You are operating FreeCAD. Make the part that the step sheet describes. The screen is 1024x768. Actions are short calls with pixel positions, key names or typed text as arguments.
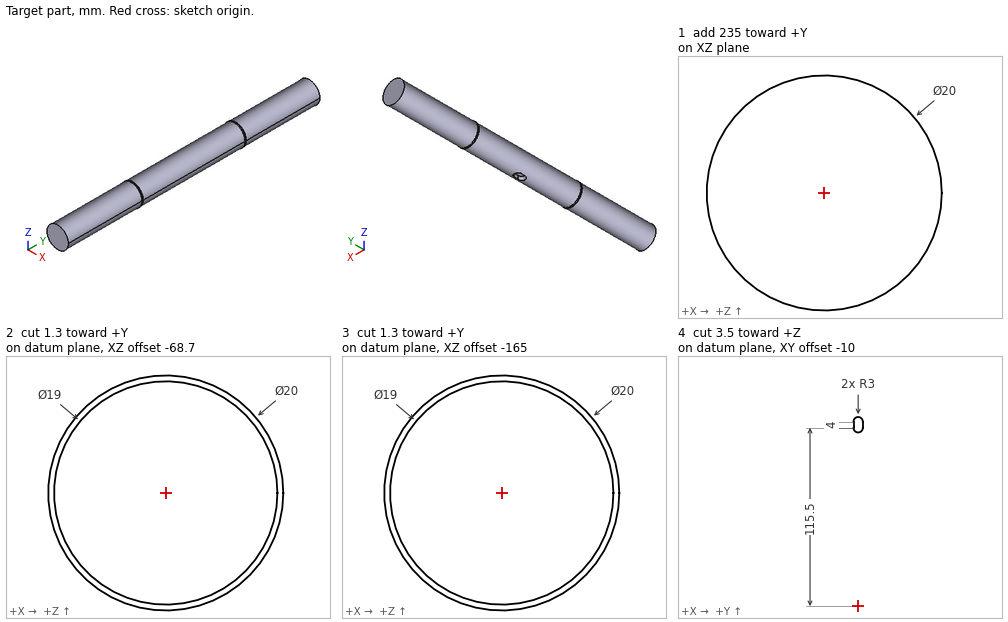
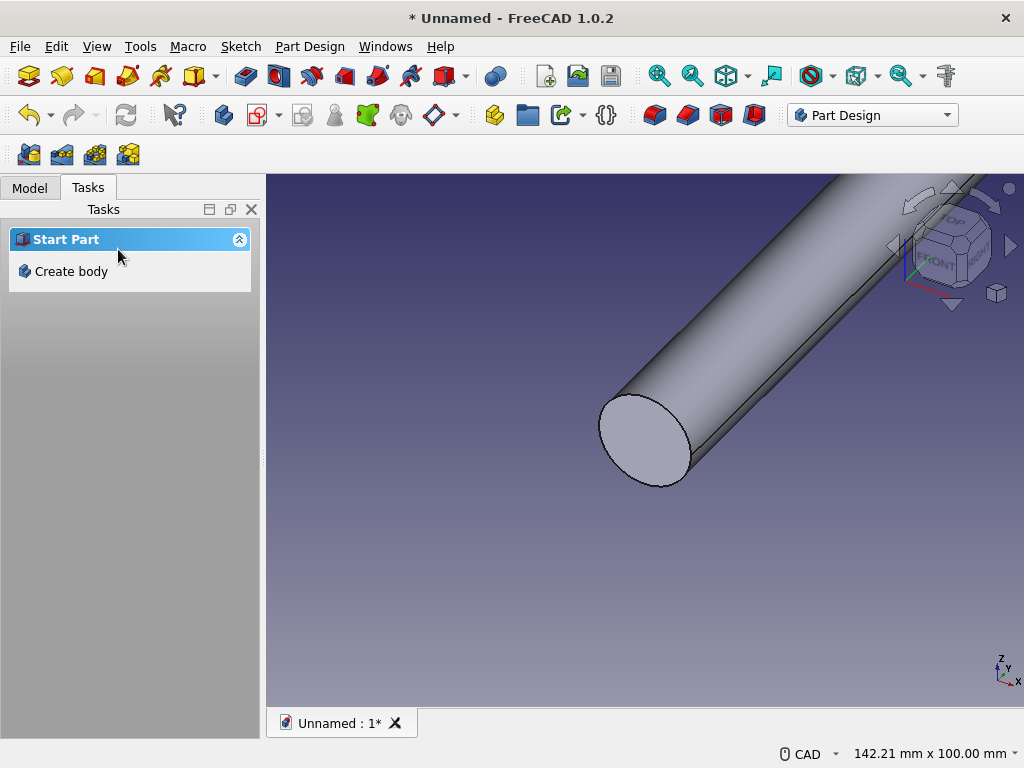
key(v)
key(f)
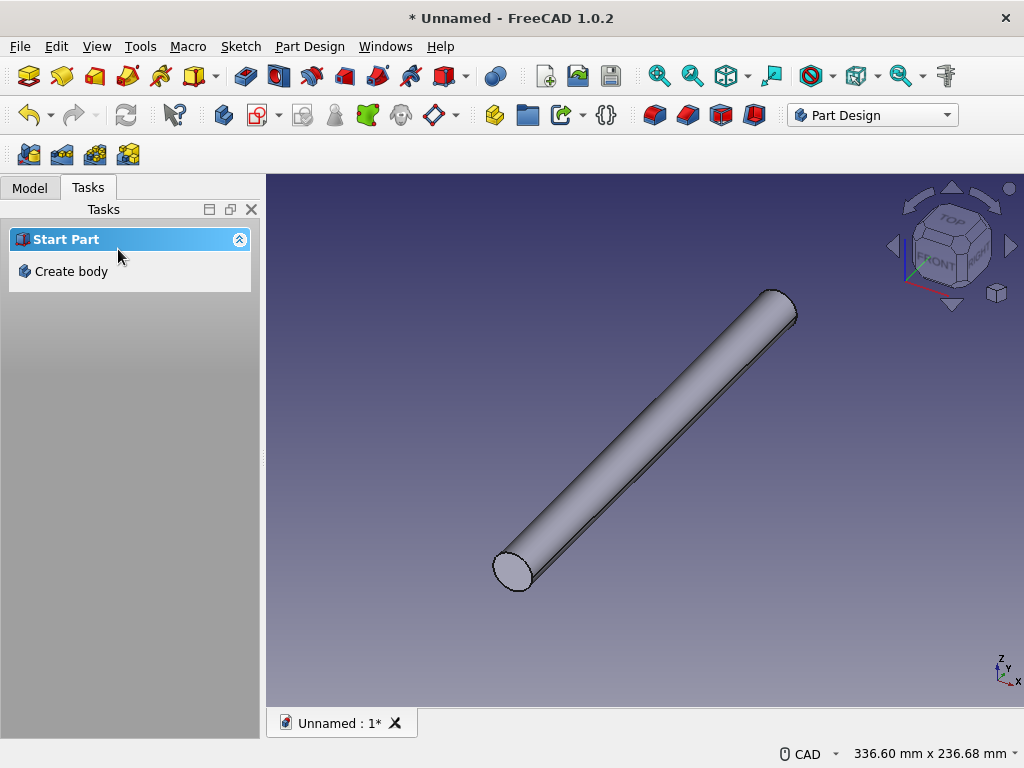
click(30, 188)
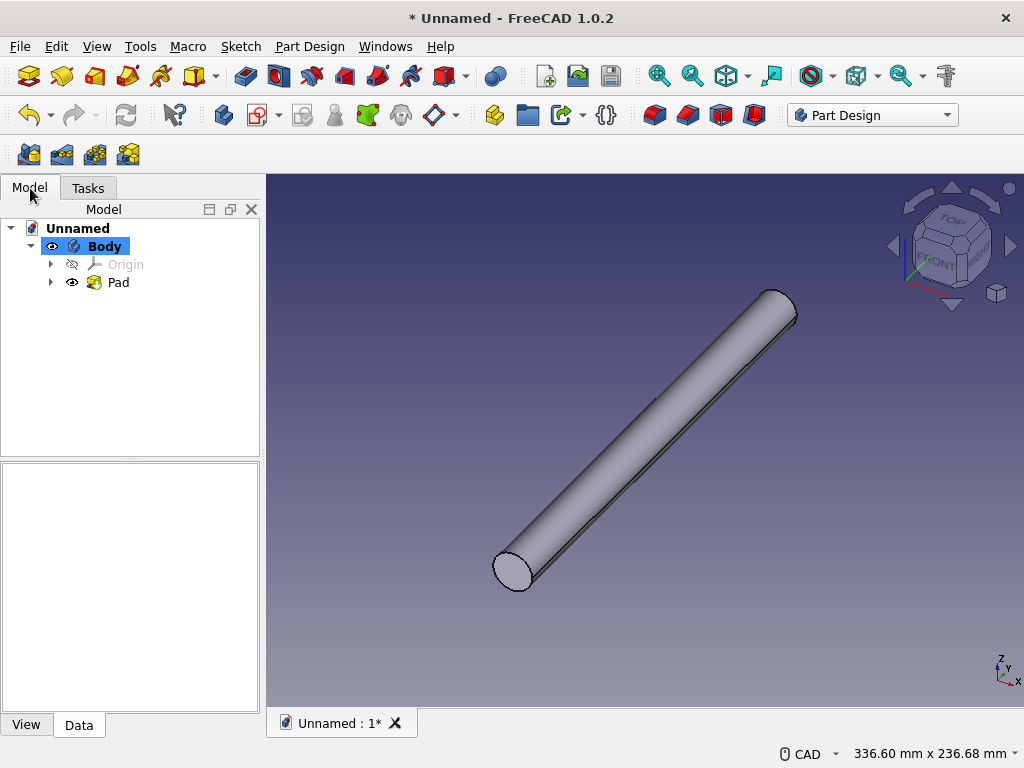
click(51, 264)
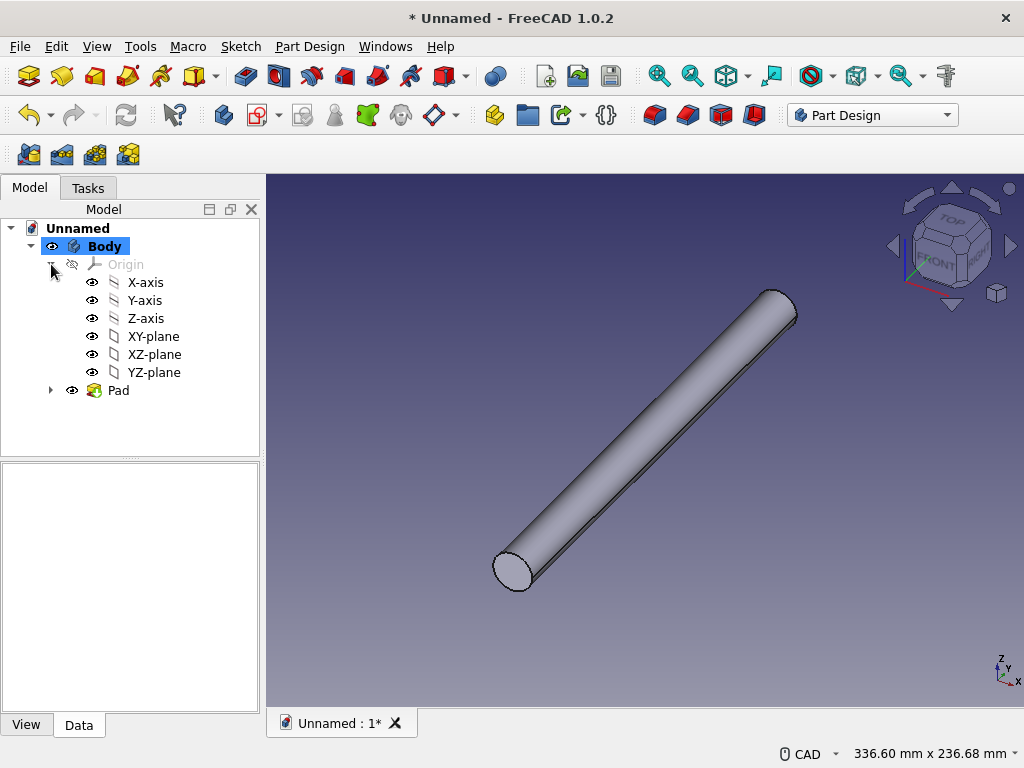
click(137, 354)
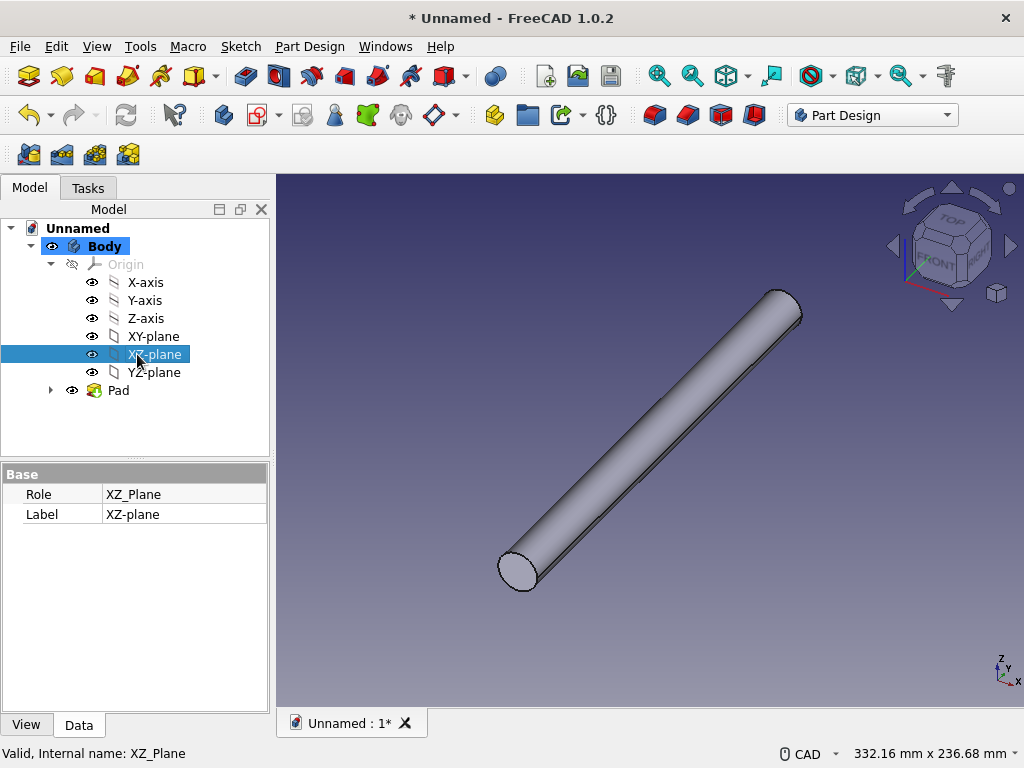
click(434, 116)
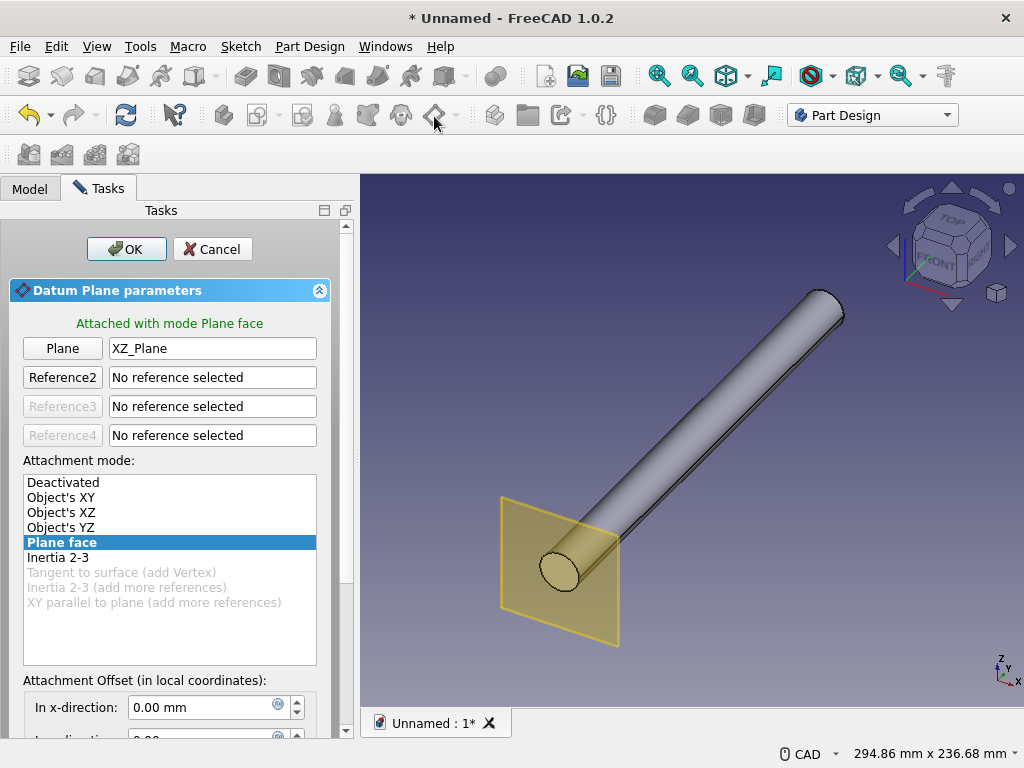
scroll(346, 479, down, 2)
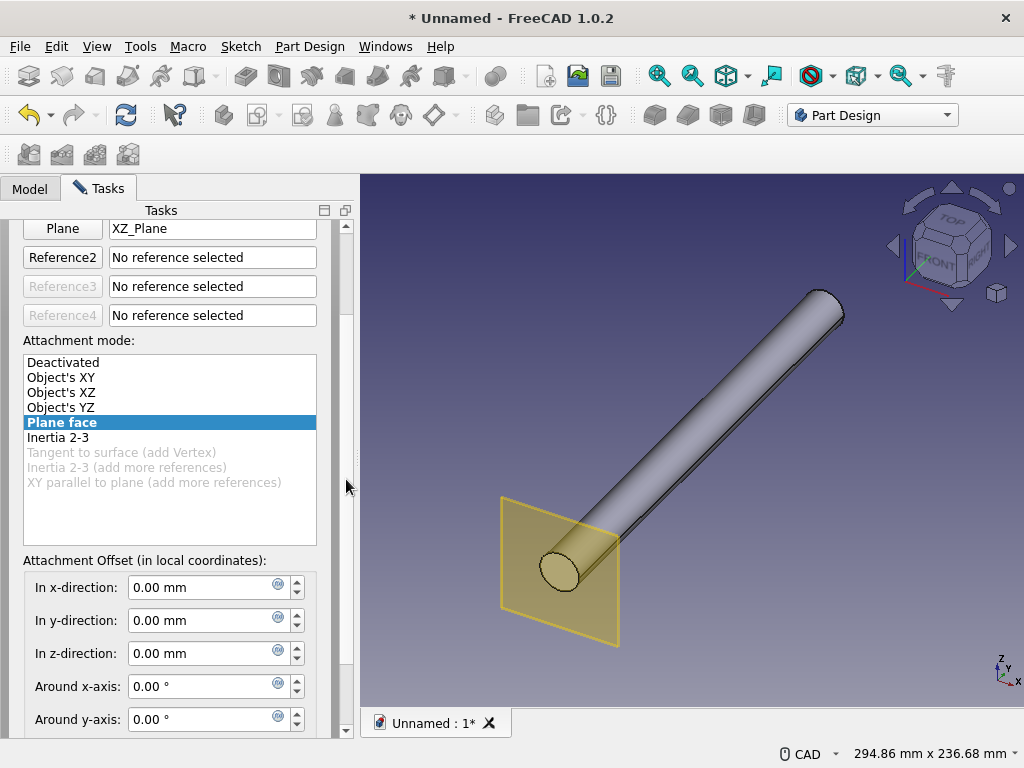
triple_click(210, 654)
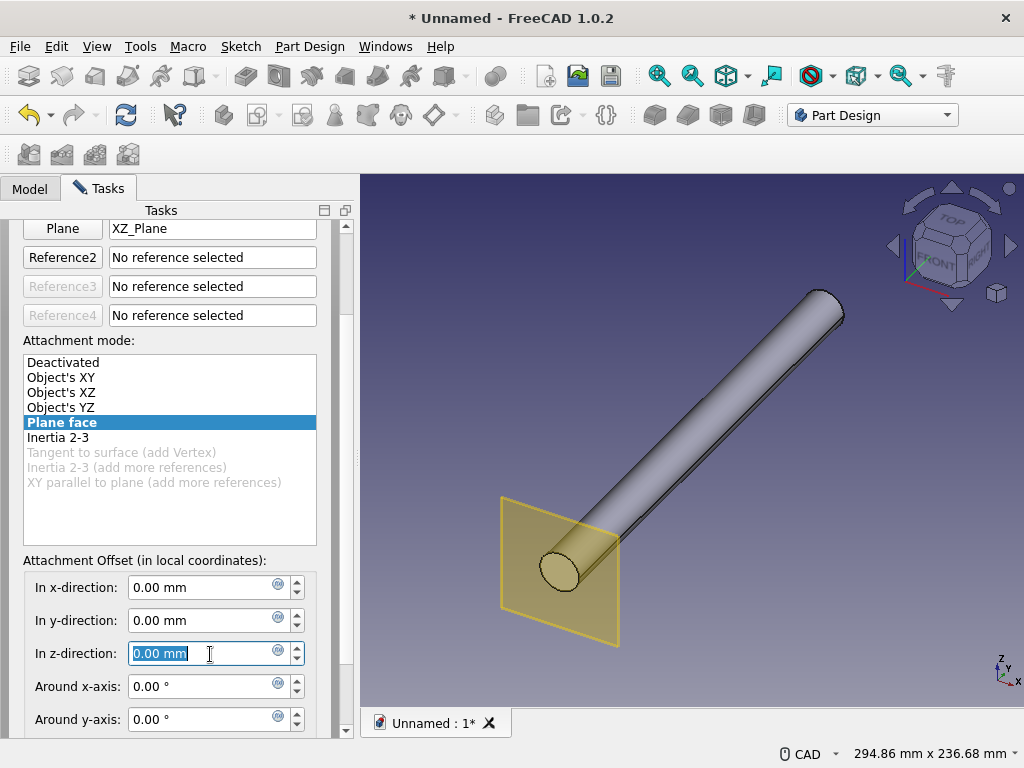
text(-68.7)
key(Tab)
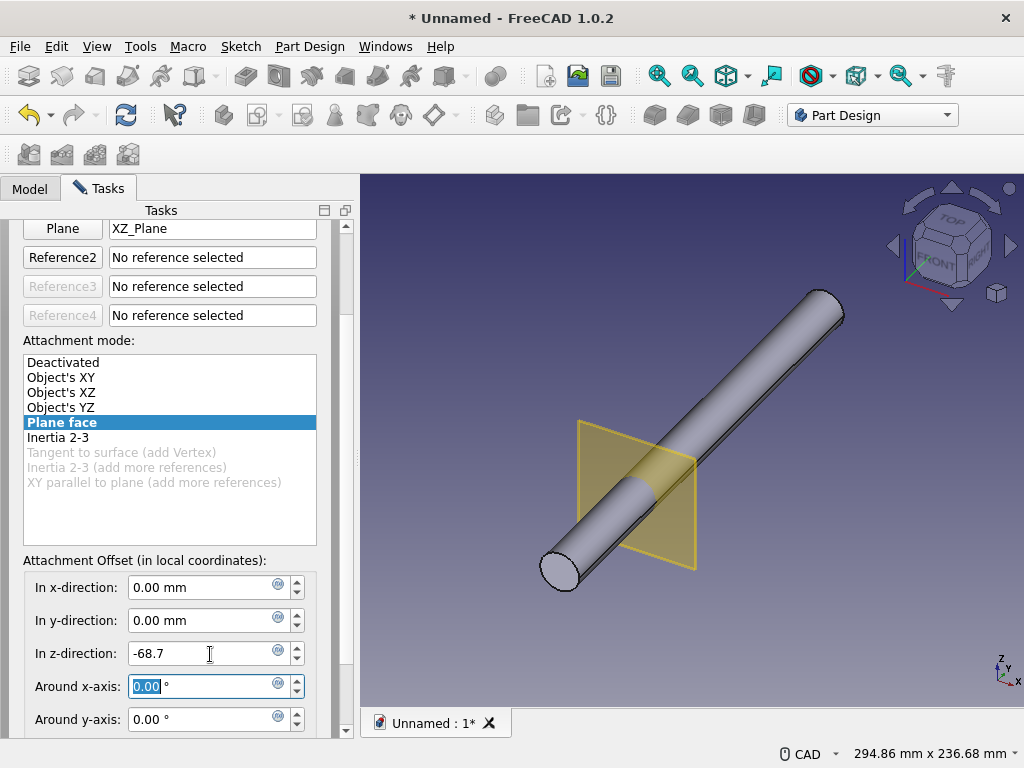
scroll(346, 479, up, 3)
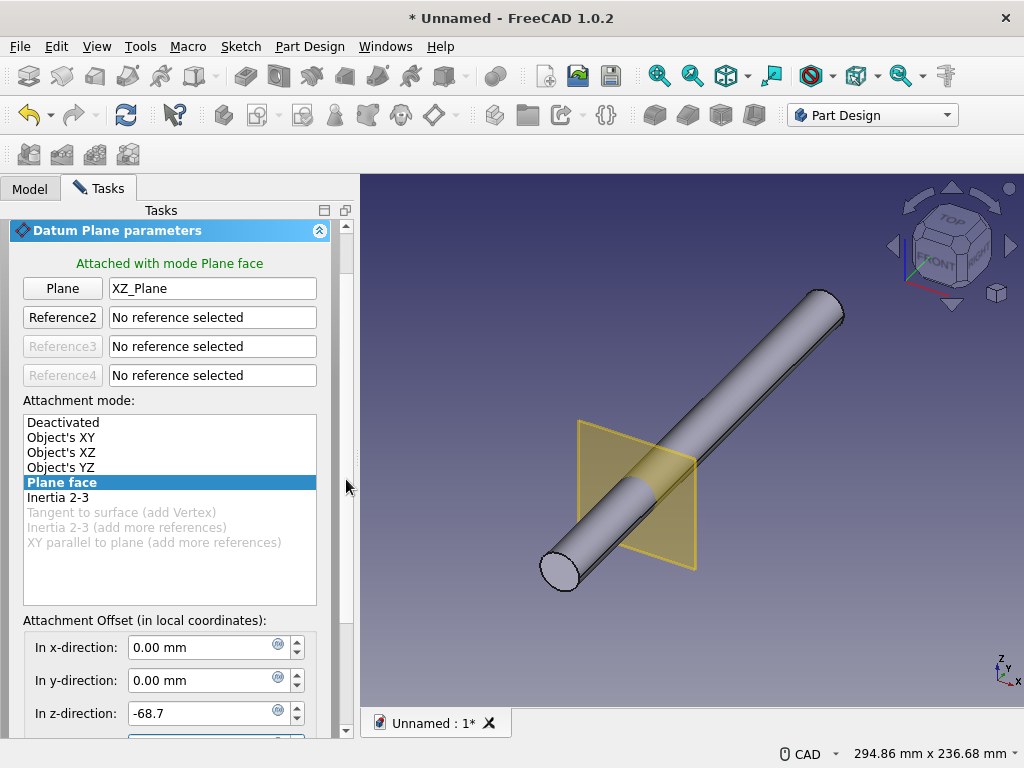
click(127, 249)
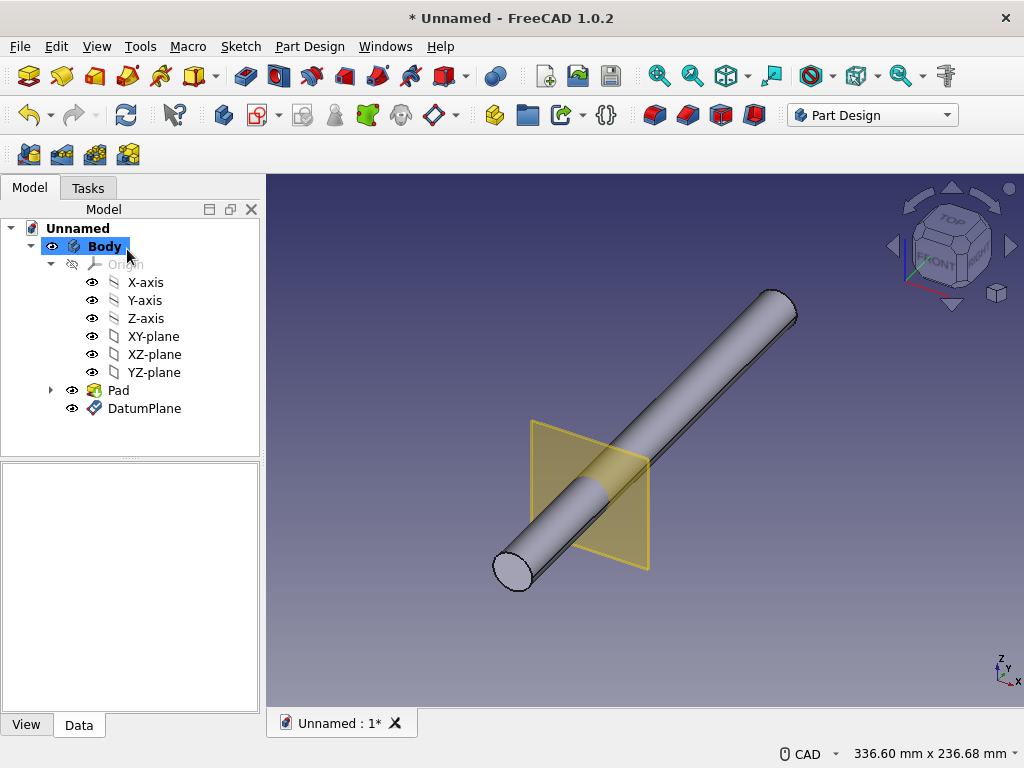
click(117, 408)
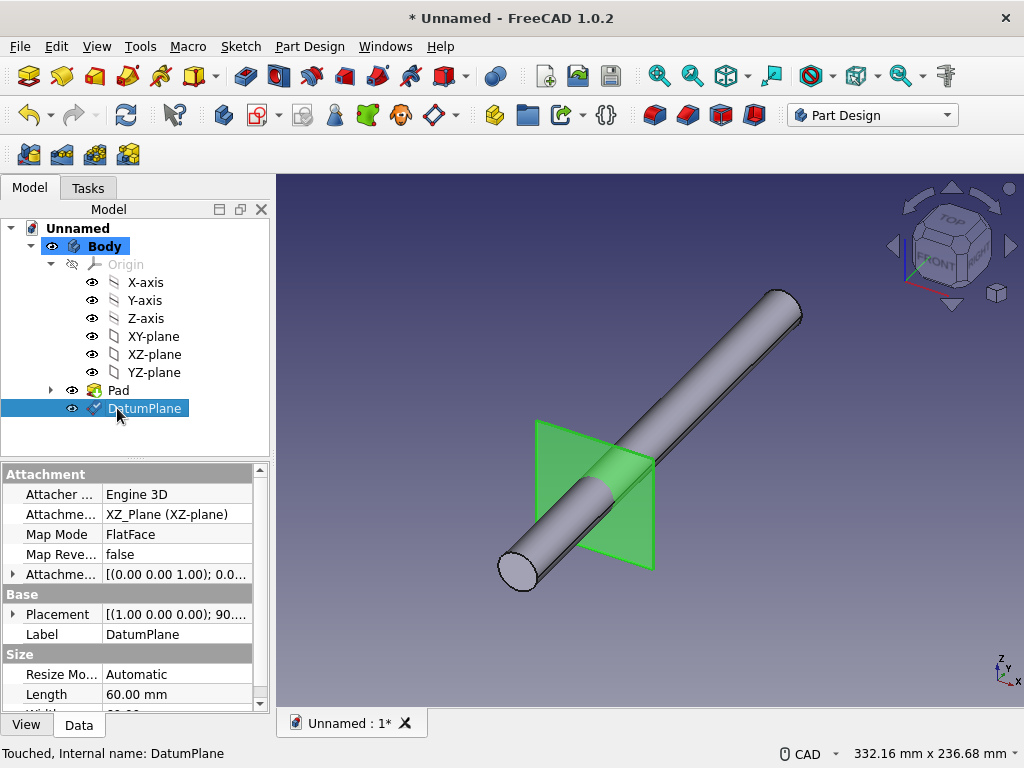
click(256, 116)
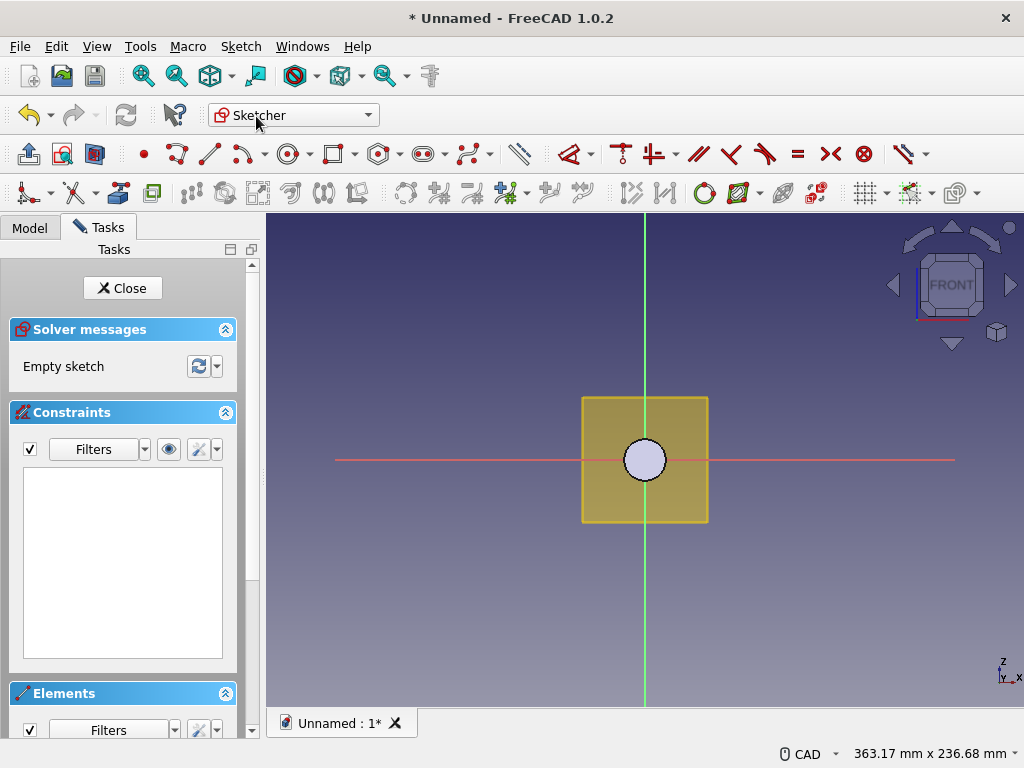
click(95, 154)